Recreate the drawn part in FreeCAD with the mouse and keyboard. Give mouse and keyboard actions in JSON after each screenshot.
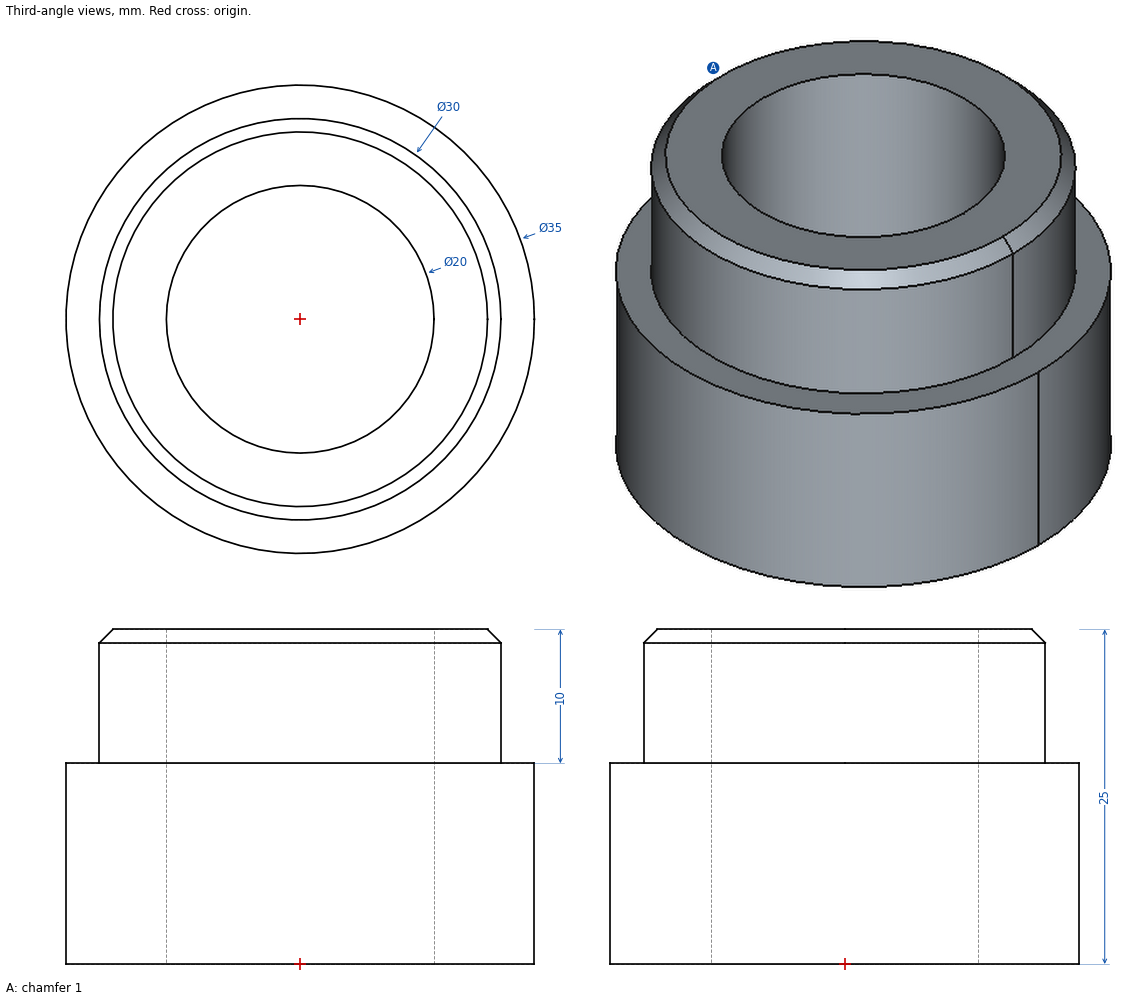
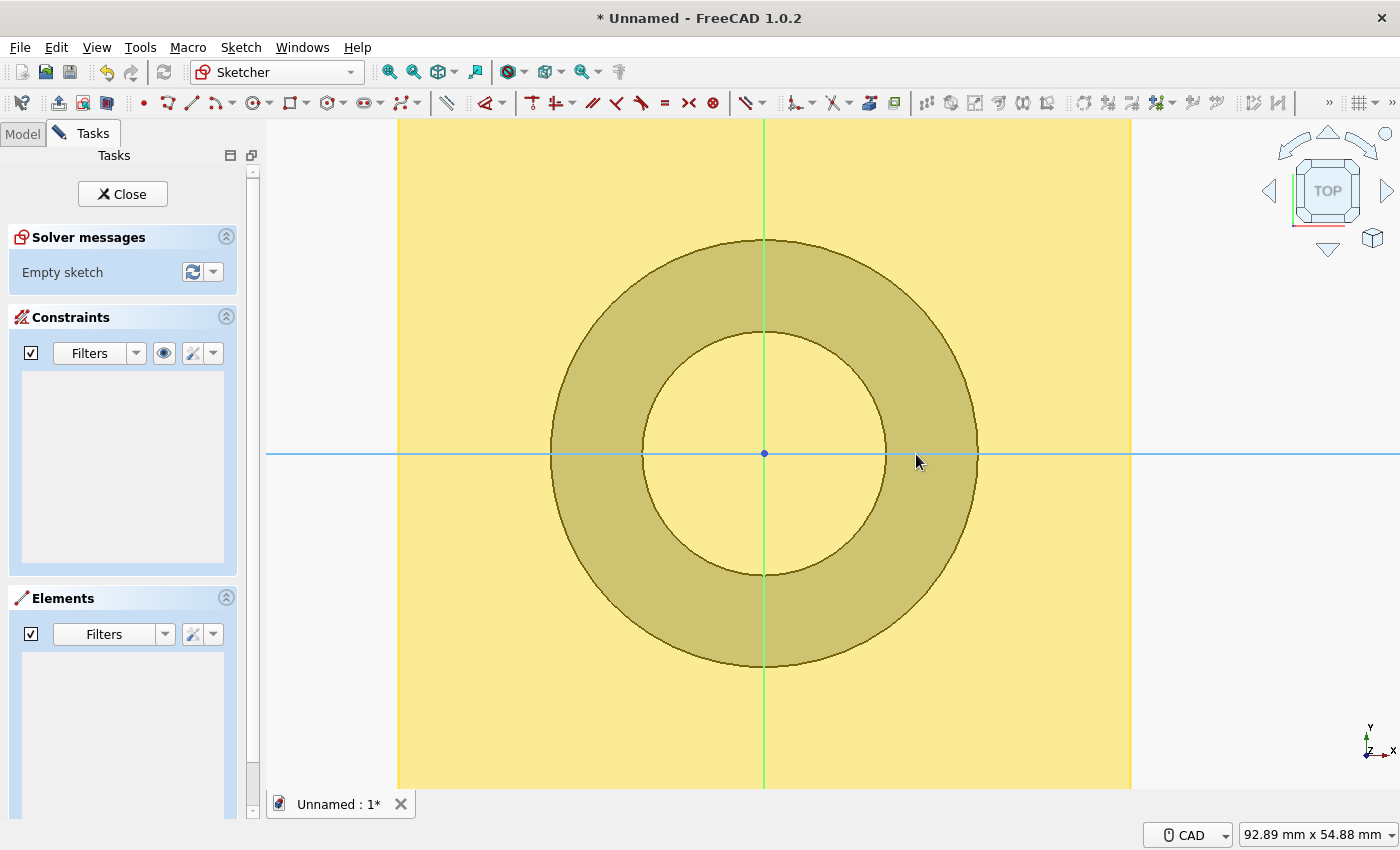
{"action": "left_click", "coordinate": [254, 104]}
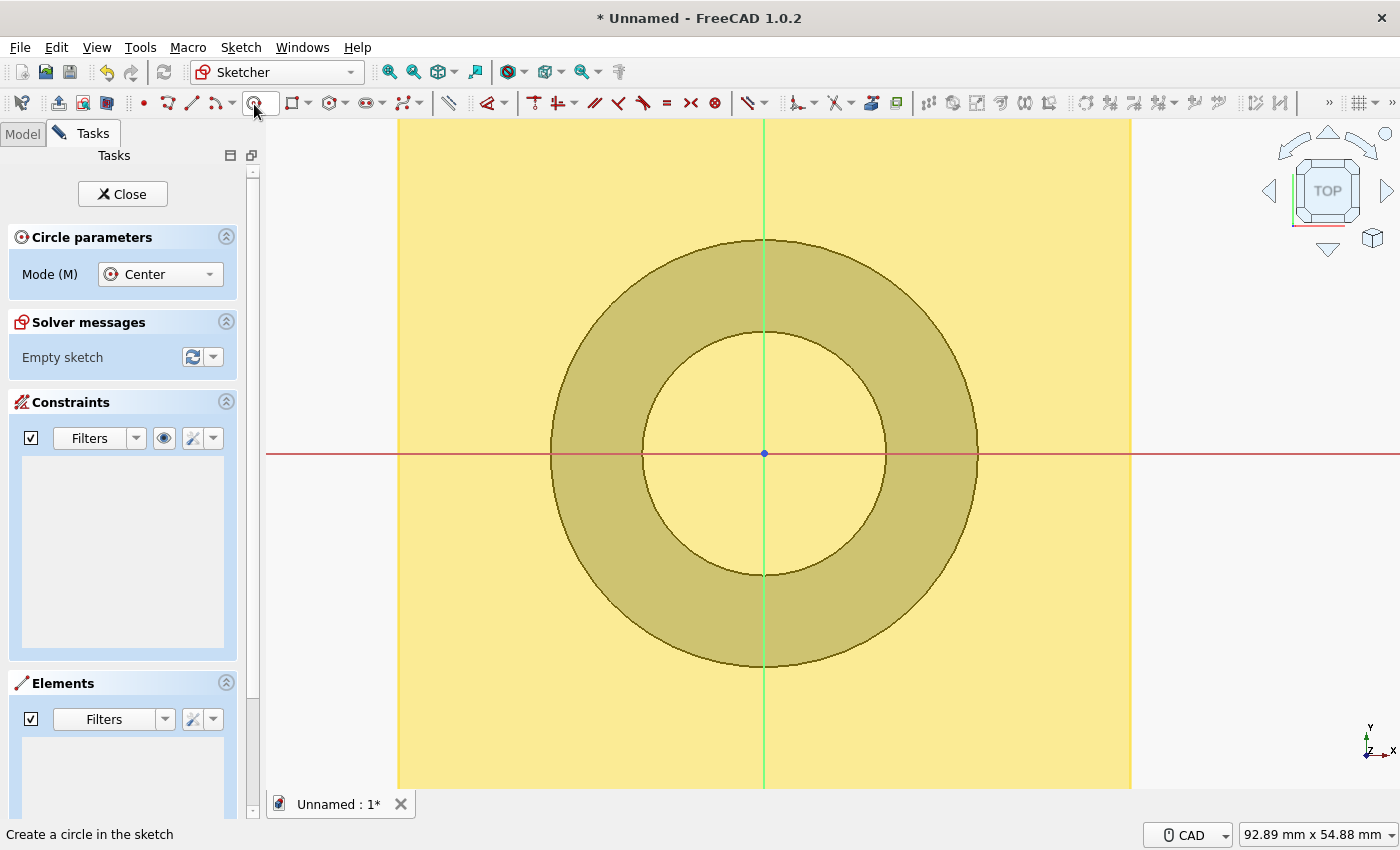
{"action": "left_click", "coordinate": [764, 454]}
{"action": "mouse_move", "coordinate": [915, 303]}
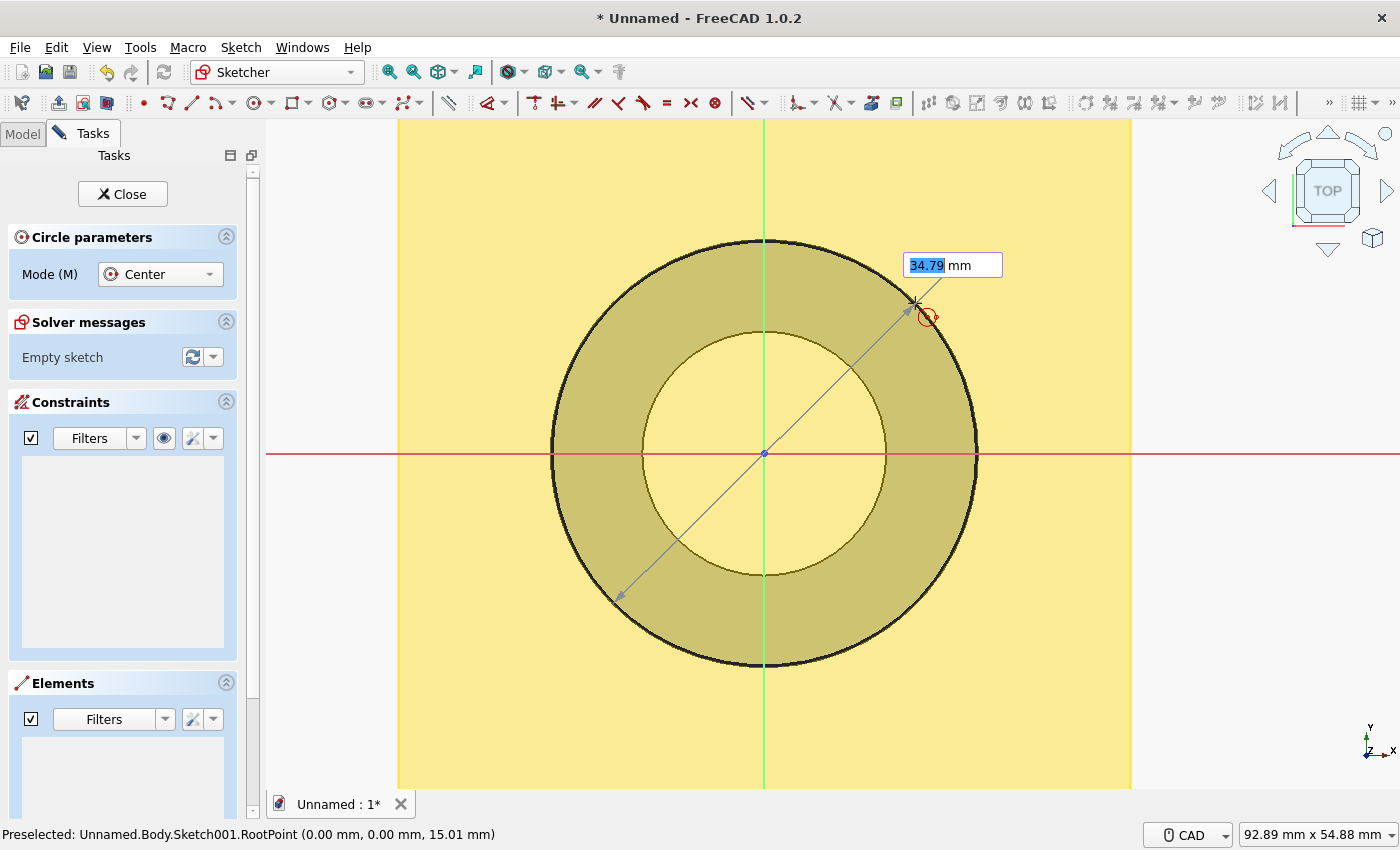
{"action": "type", "text": "35"}
{"action": "key", "text": "Return"}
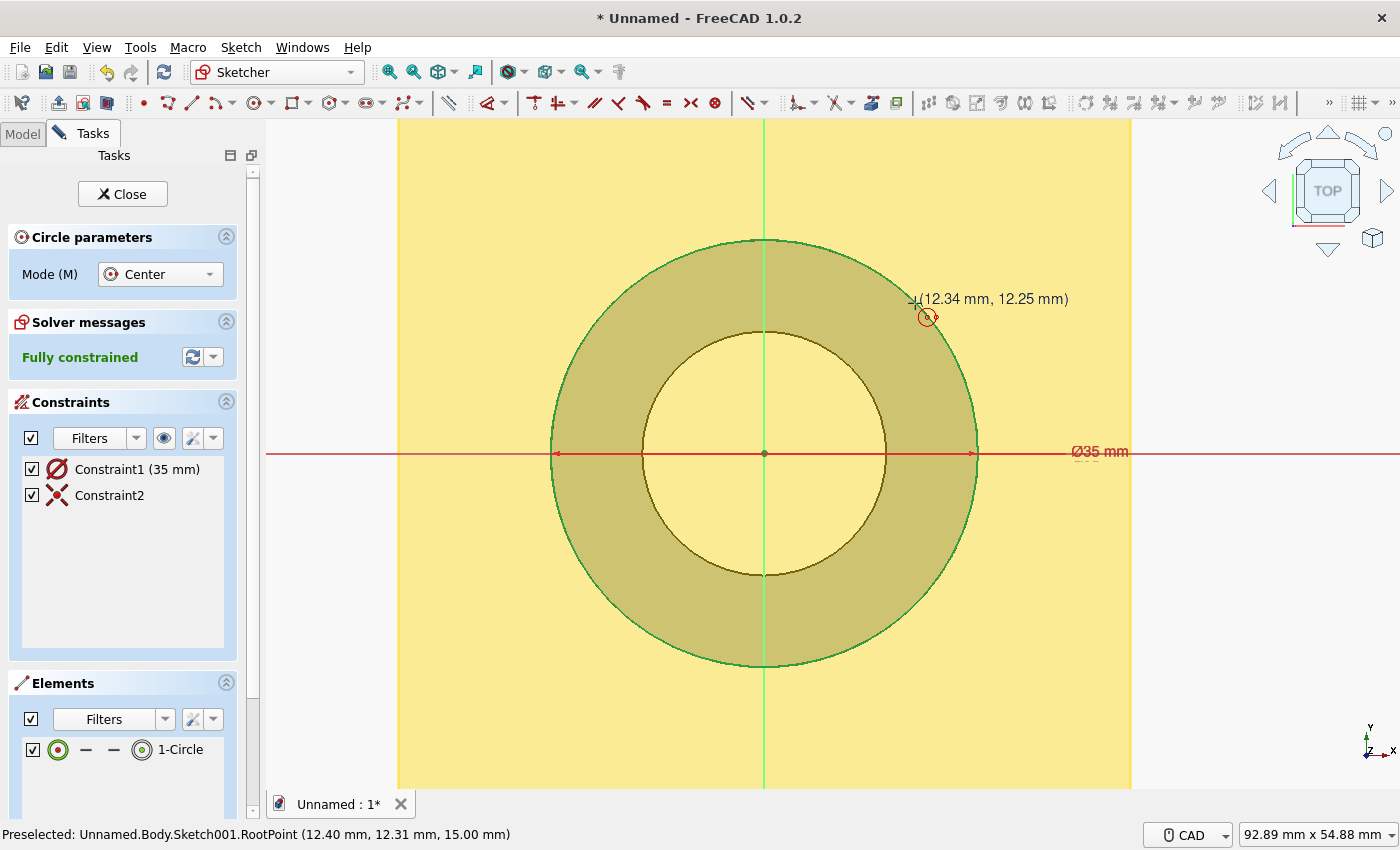
{"action": "left_click", "coordinate": [764, 454]}
{"action": "mouse_move", "coordinate": [894, 324]}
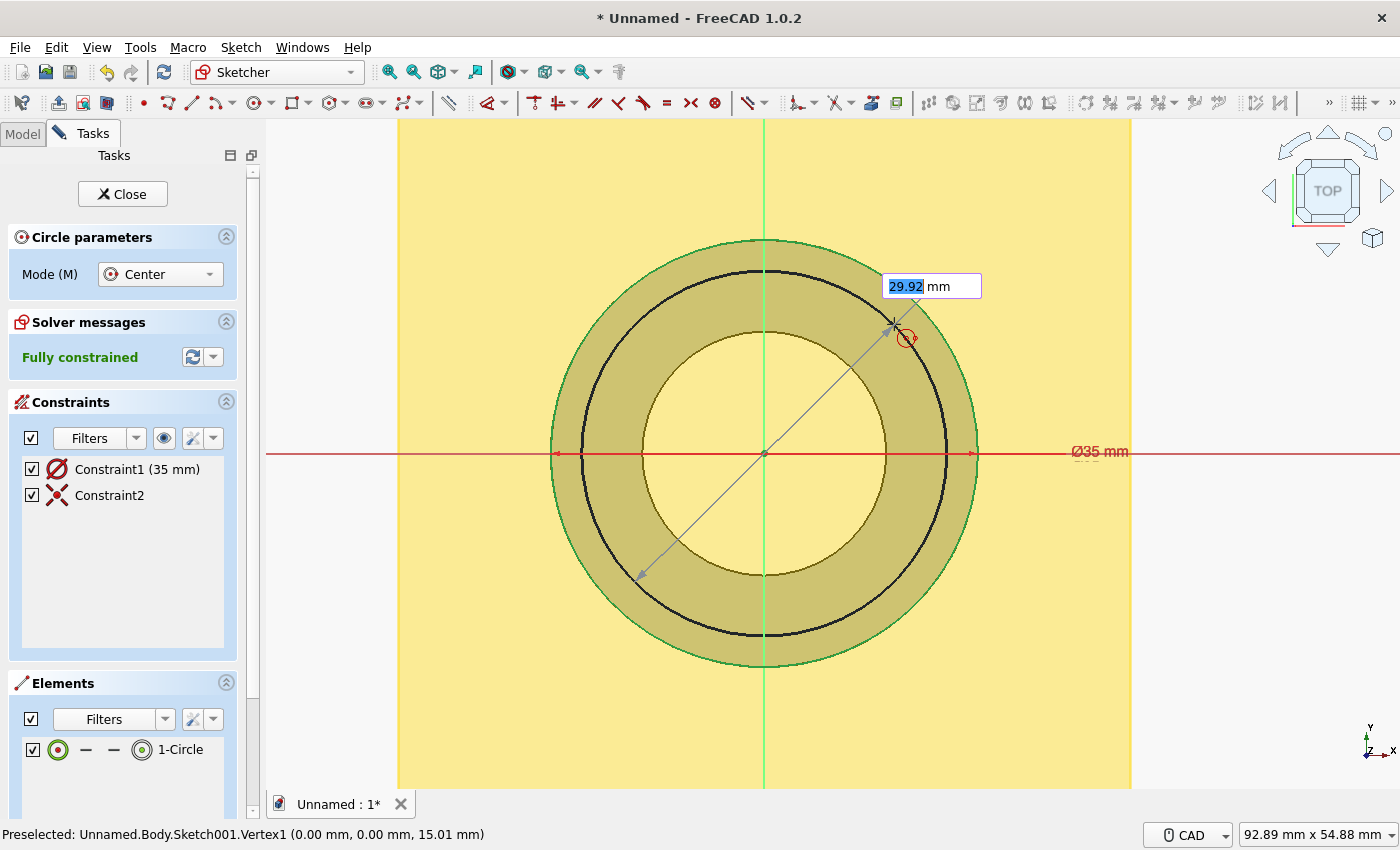
{"action": "type", "text": "30"}
{"action": "key", "text": "Return"}
{"action": "key", "text": "Escape"}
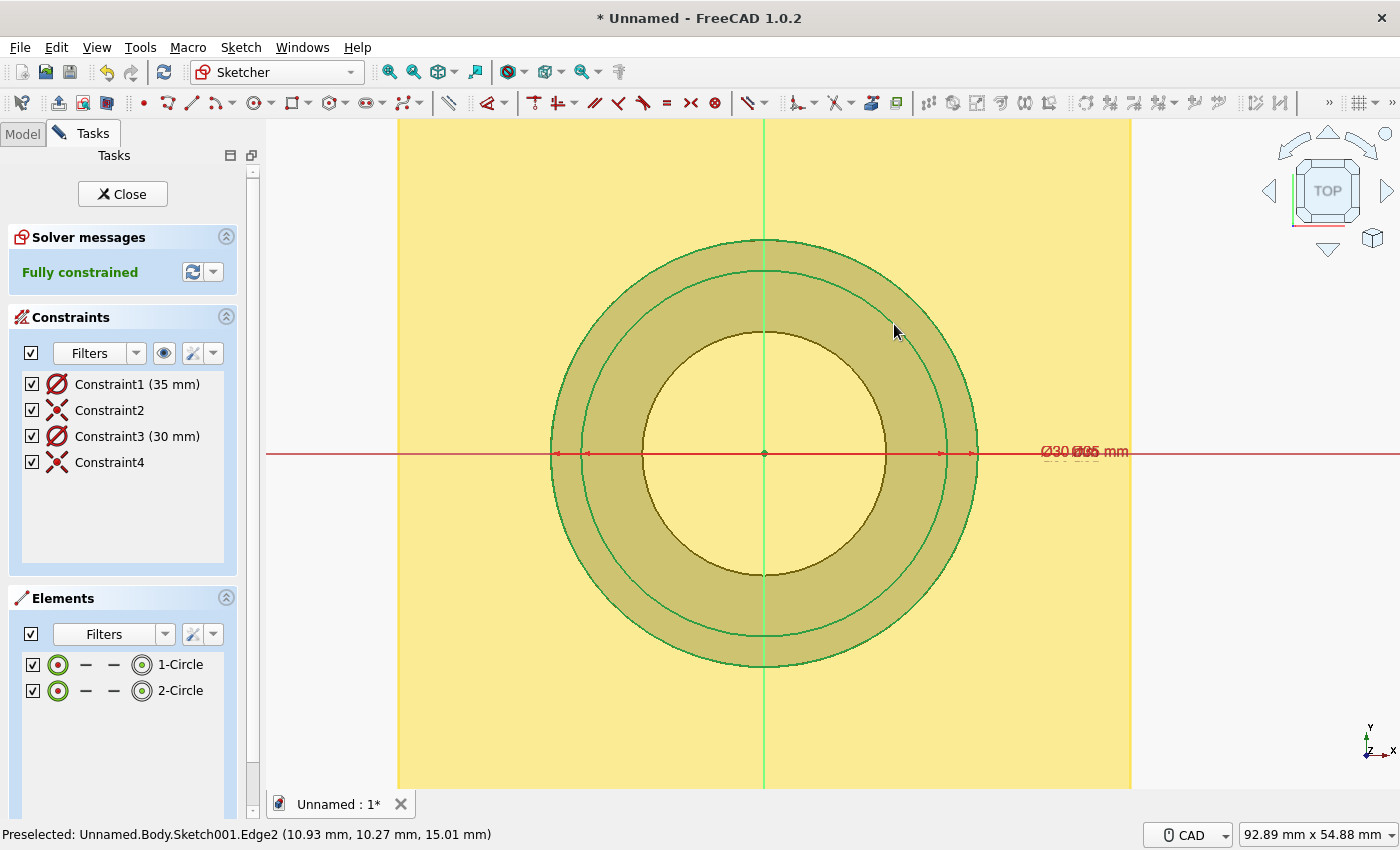
{"action": "left_click", "coordinate": [123, 194]}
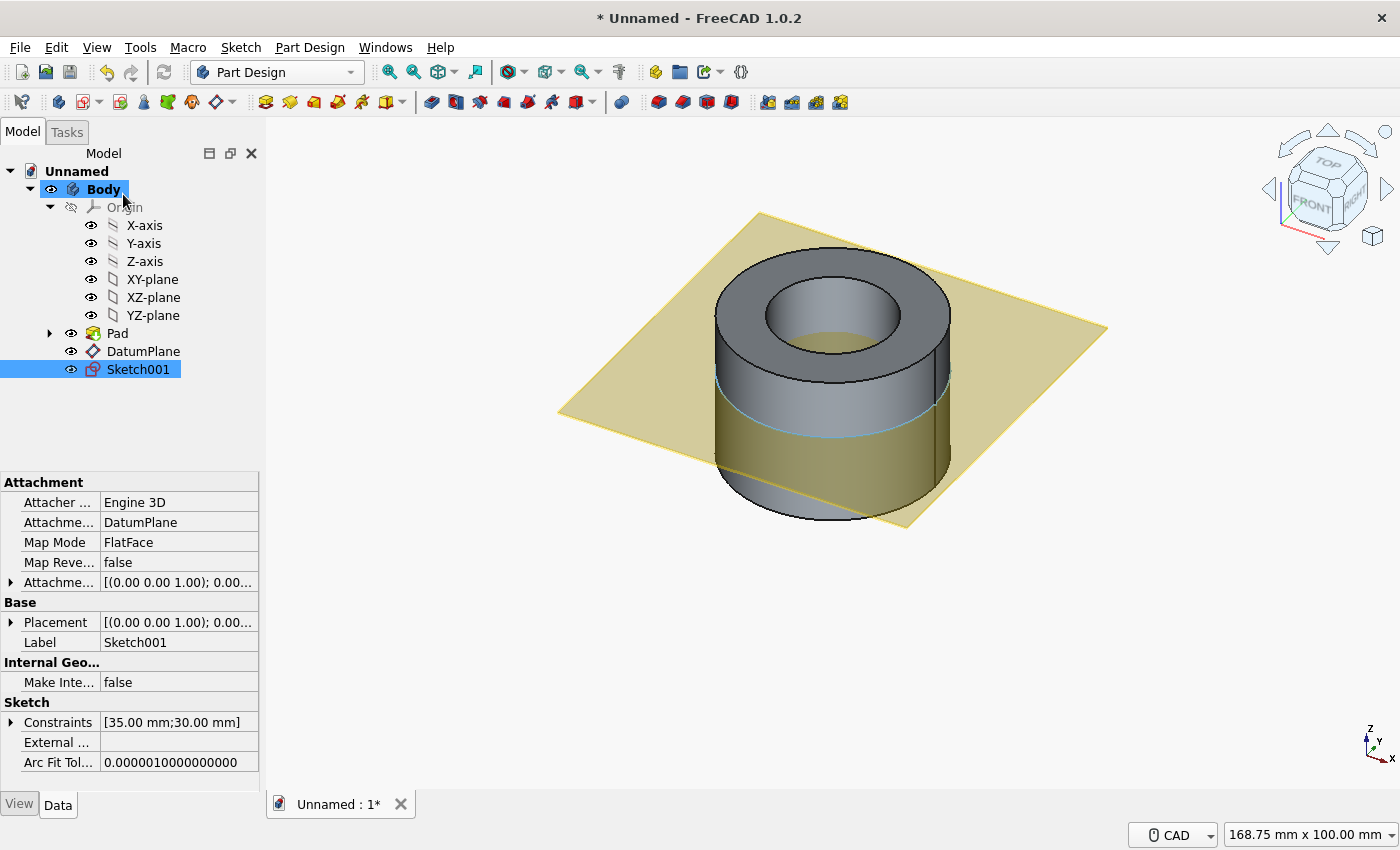
{"action": "left_click", "coordinate": [432, 102]}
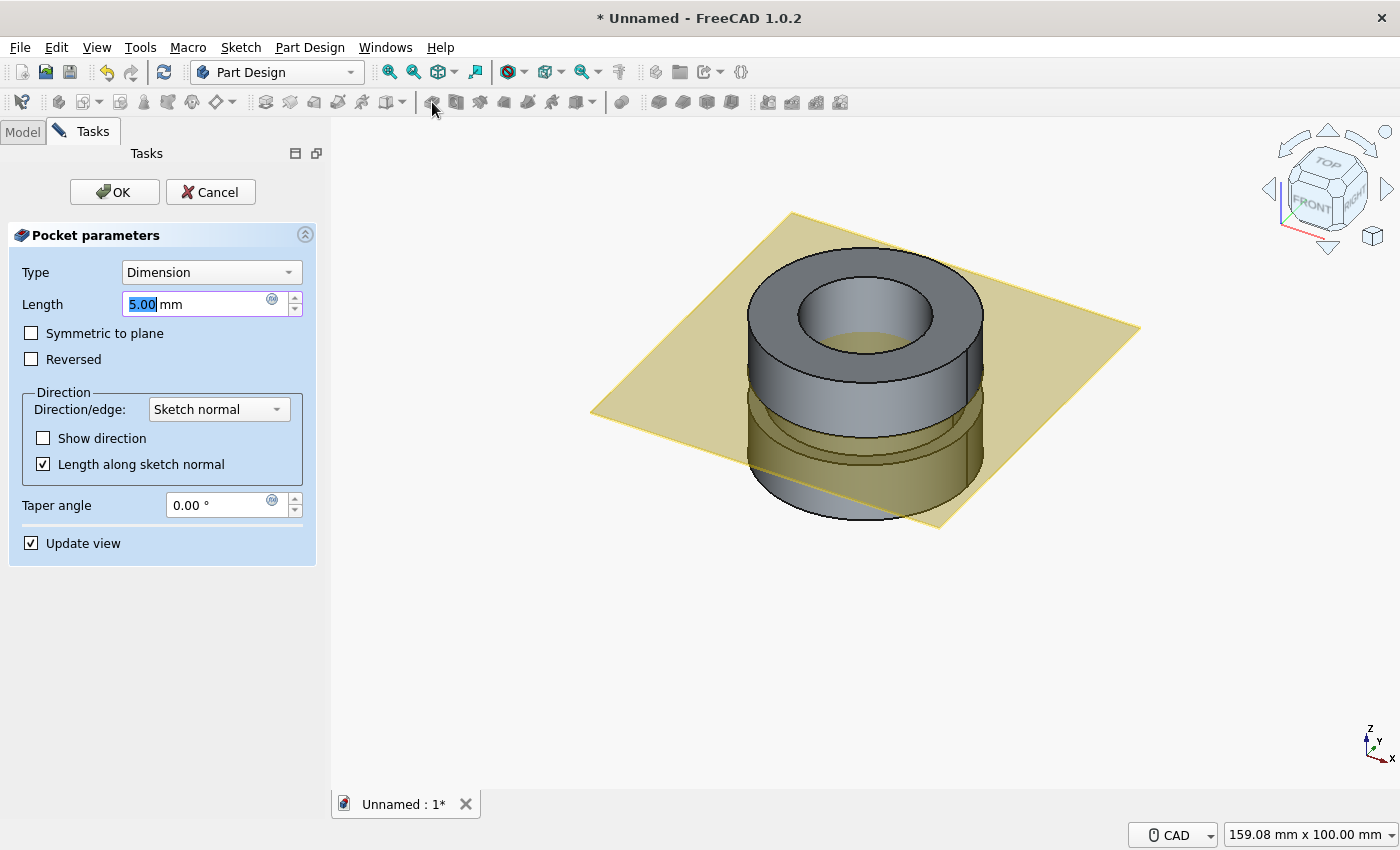
{"action": "type", "text": "10"}
{"action": "key", "text": "Tab"}